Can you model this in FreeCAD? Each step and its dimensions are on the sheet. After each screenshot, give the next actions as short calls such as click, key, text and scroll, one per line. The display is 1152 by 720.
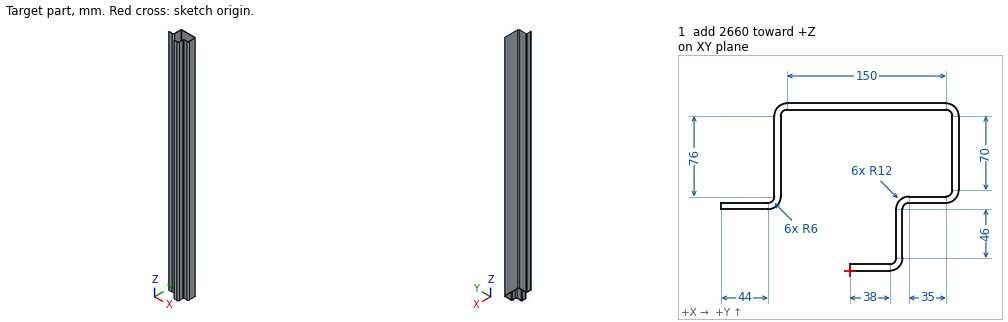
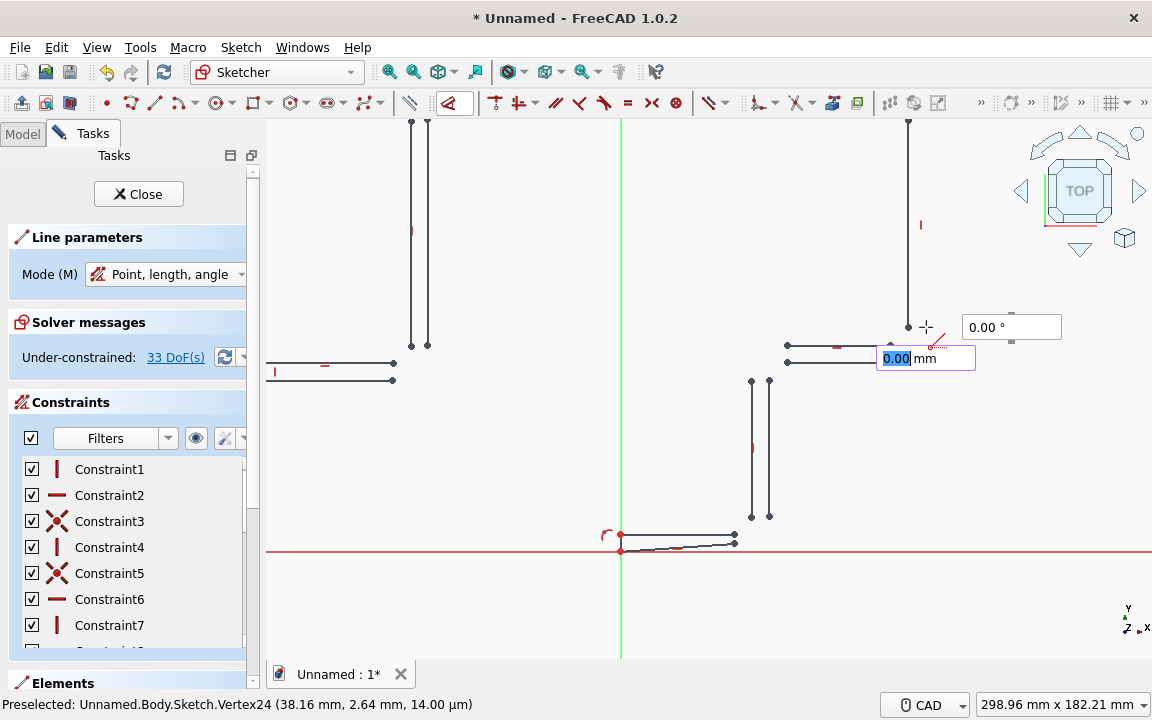
scroll(735, 534, down, 2)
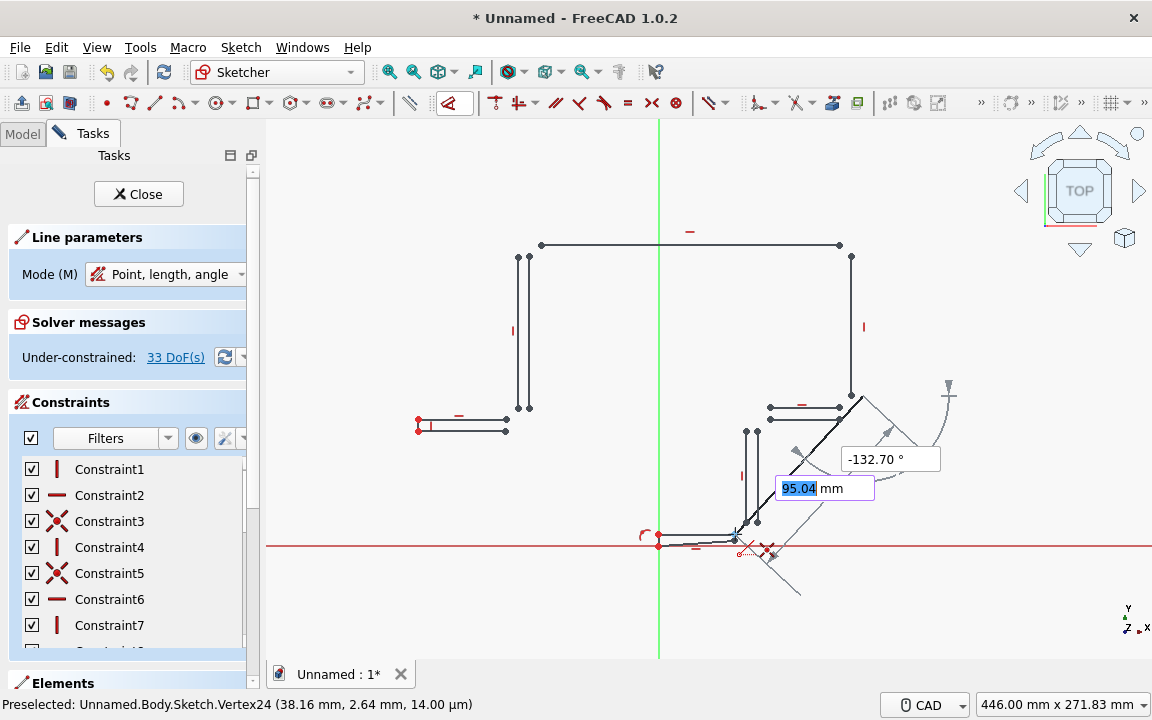
scroll(863, 256, up, 2)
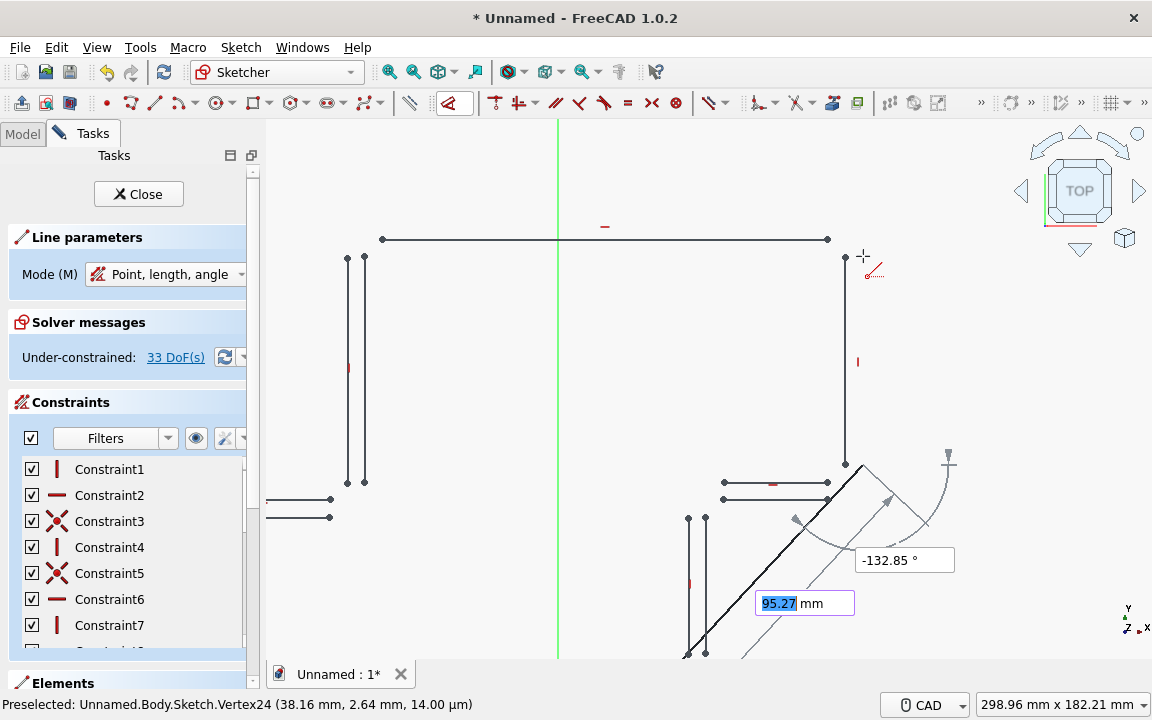
click(863, 256)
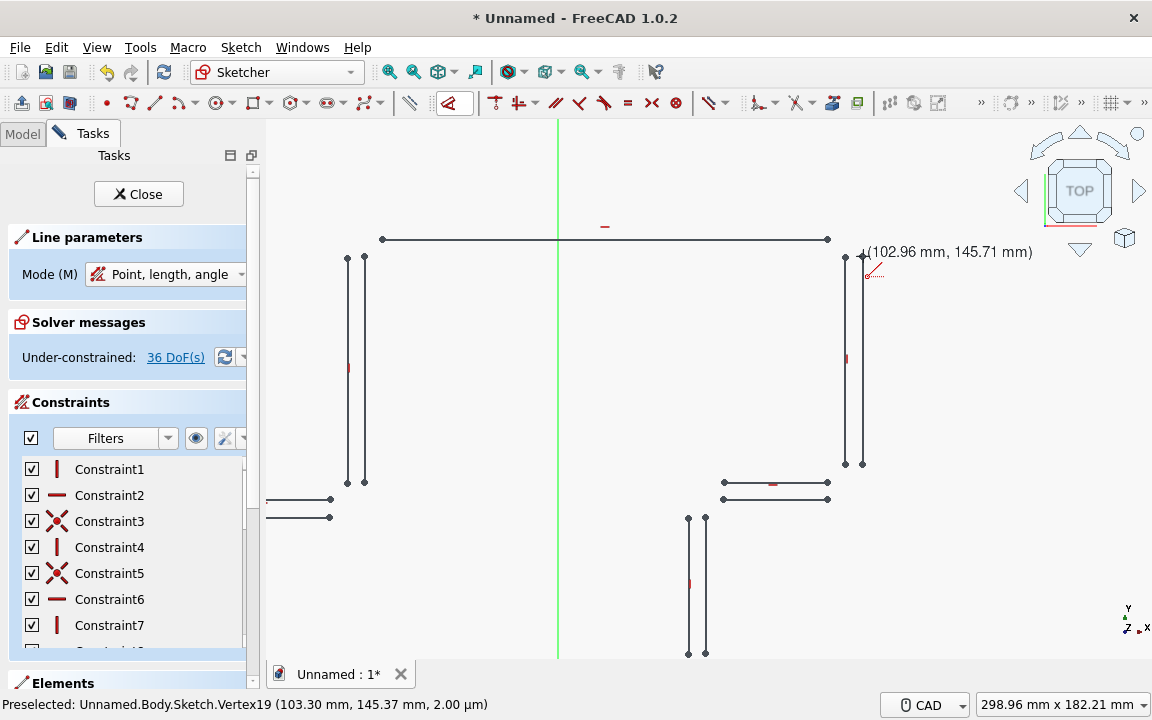
click(828, 221)
click(383, 221)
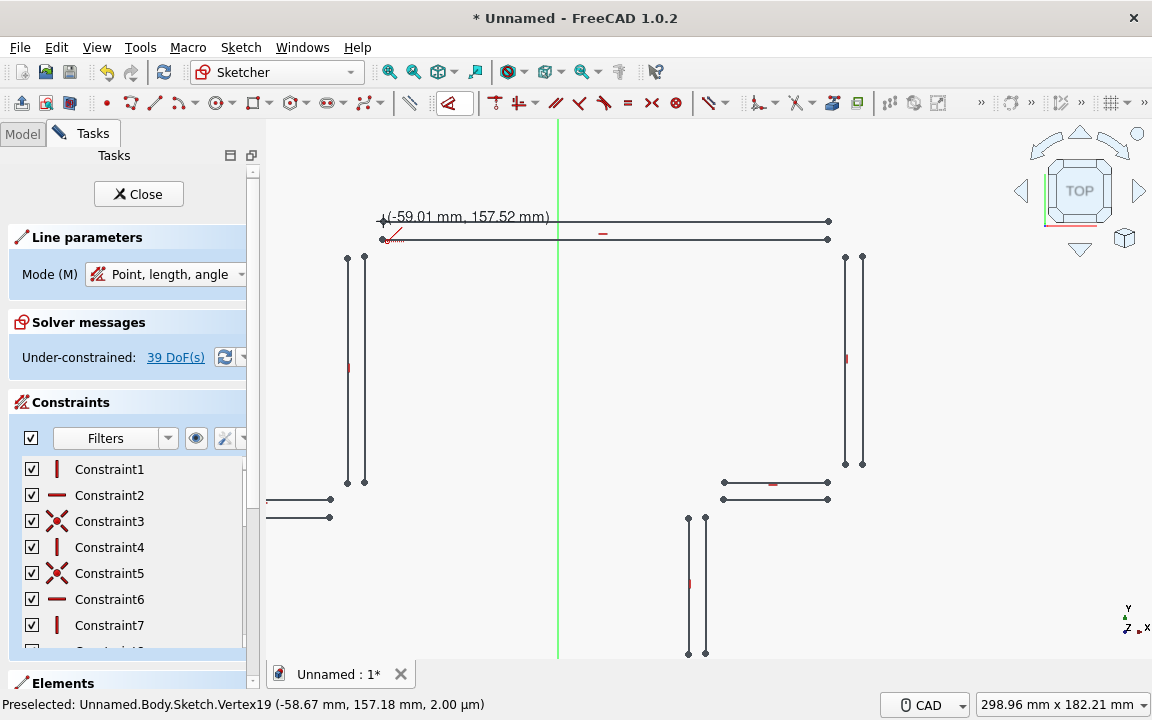
key(g)
key(3)
key(a)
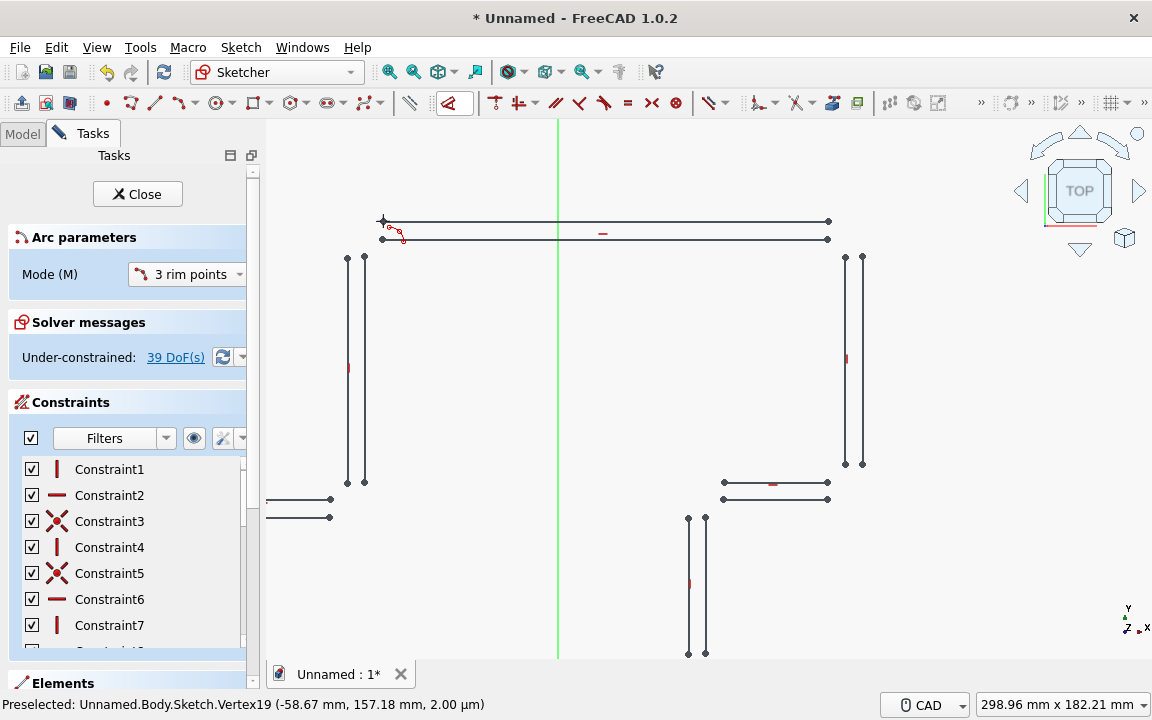
click(348, 484)
click(330, 500)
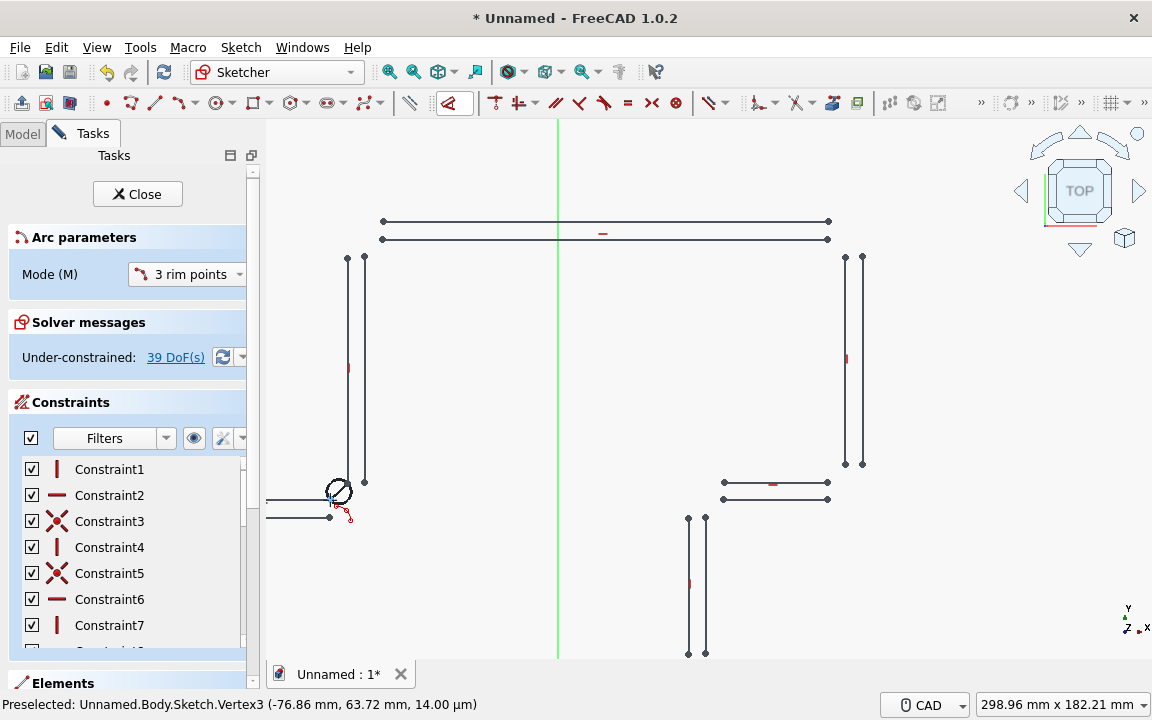
scroll(342, 494, up, 6)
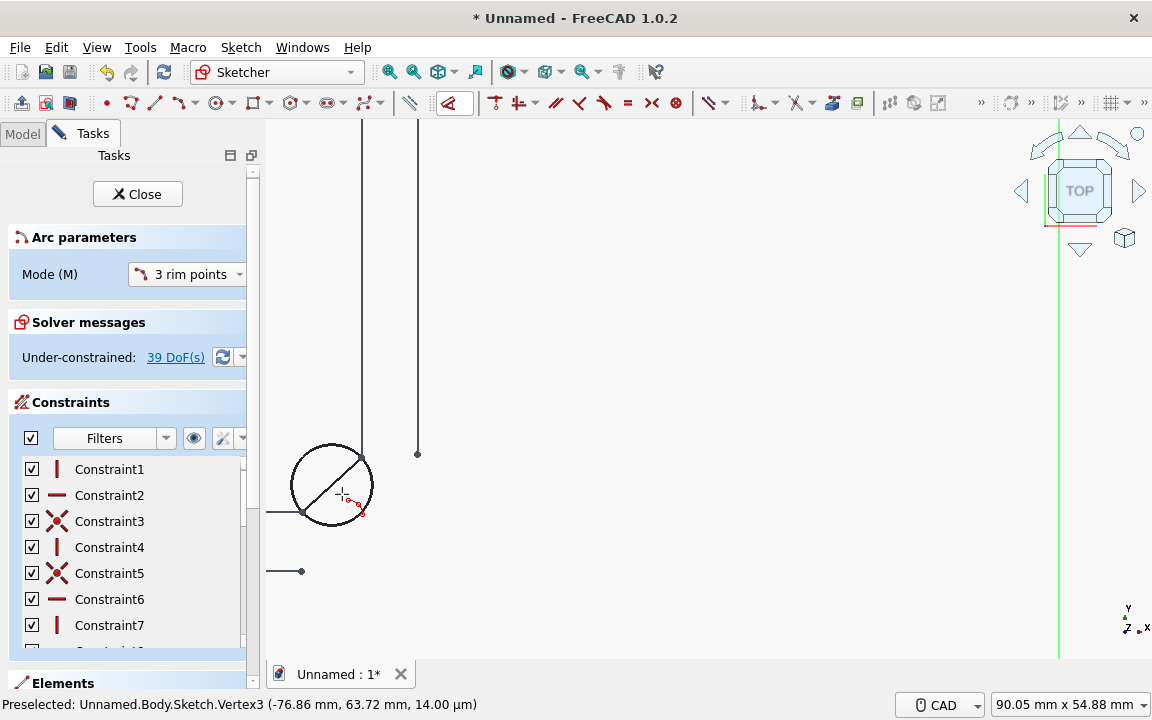
click(343, 492)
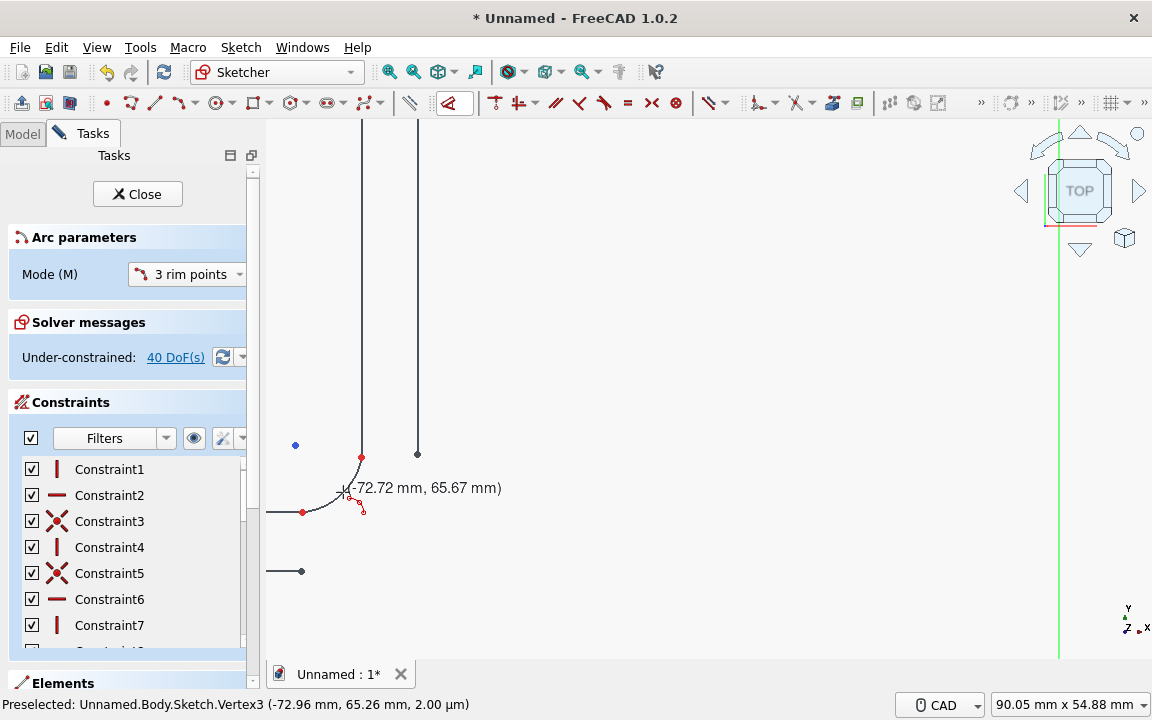
scroll(557, 396, down, 8)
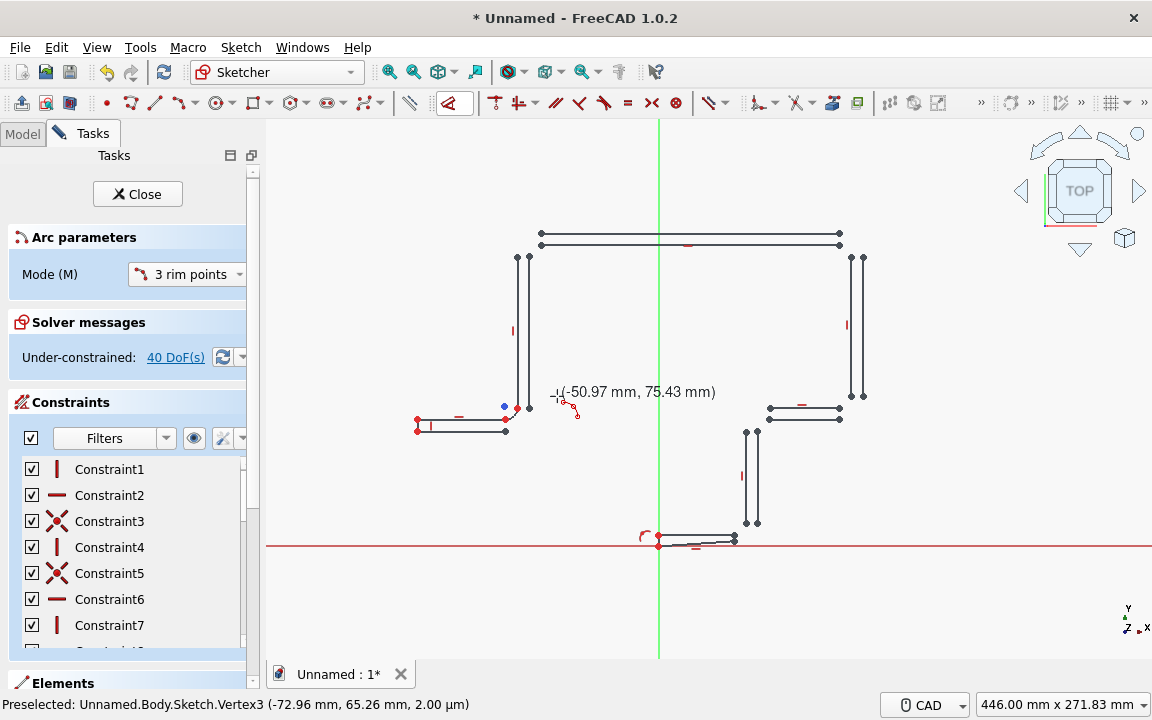
scroll(506, 431, up, 2)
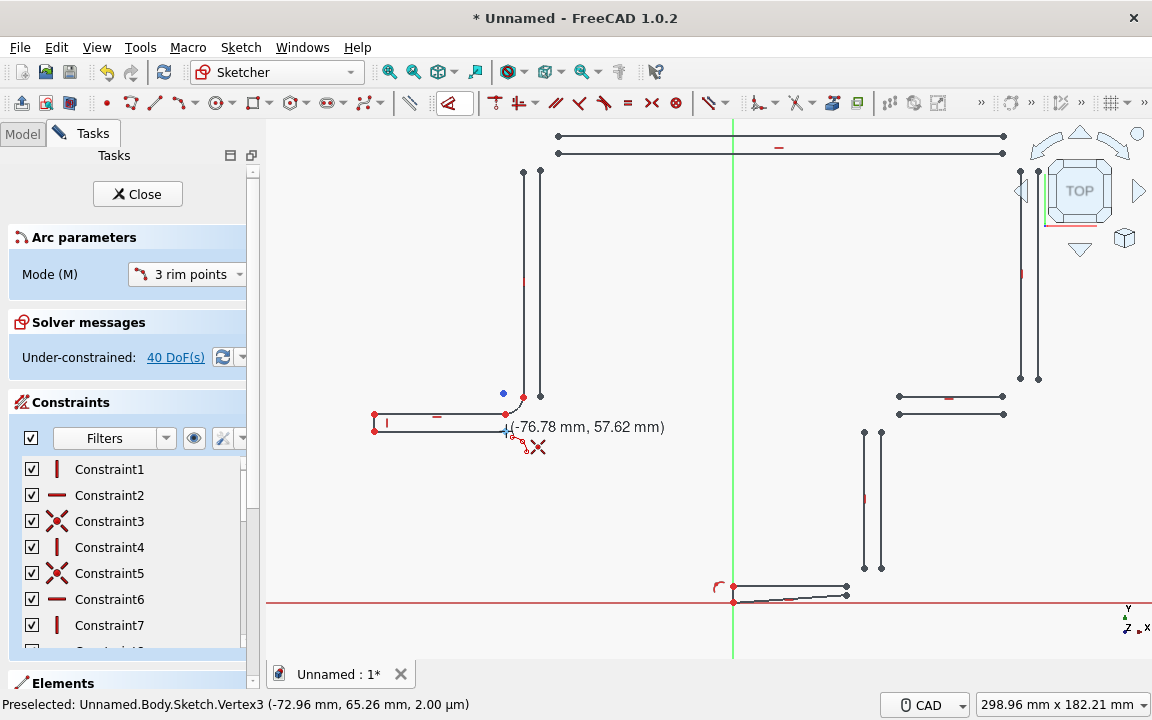
click(505, 432)
click(540, 397)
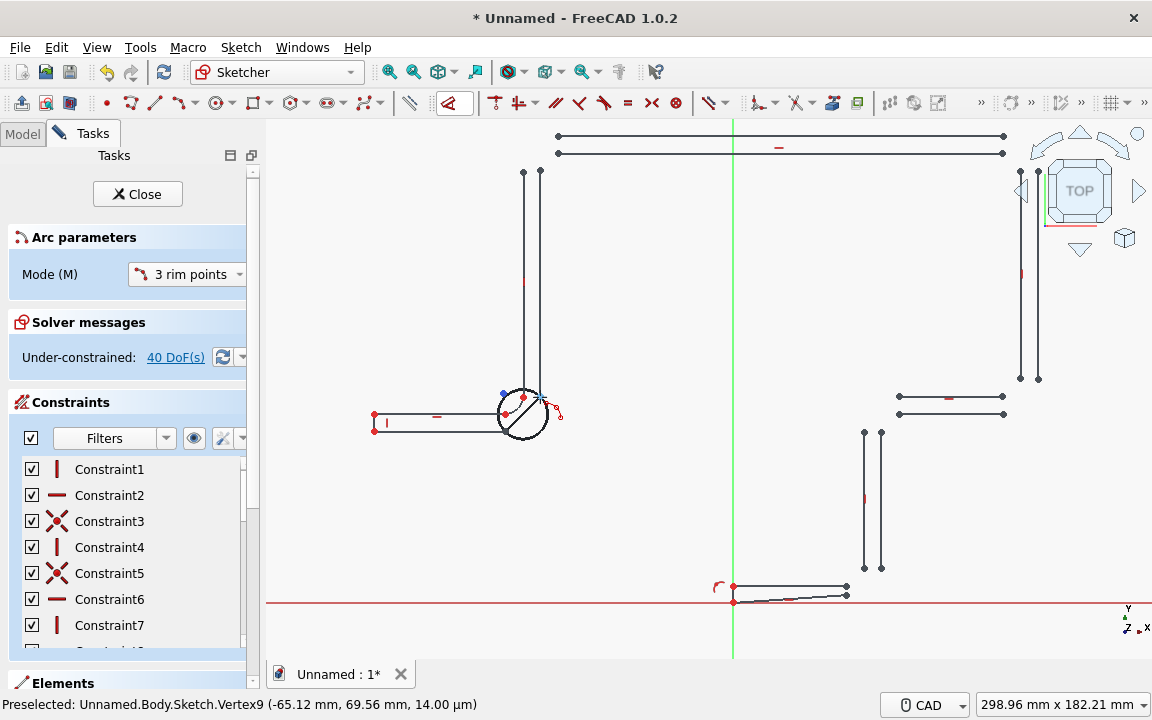
scroll(530, 421, up, 3)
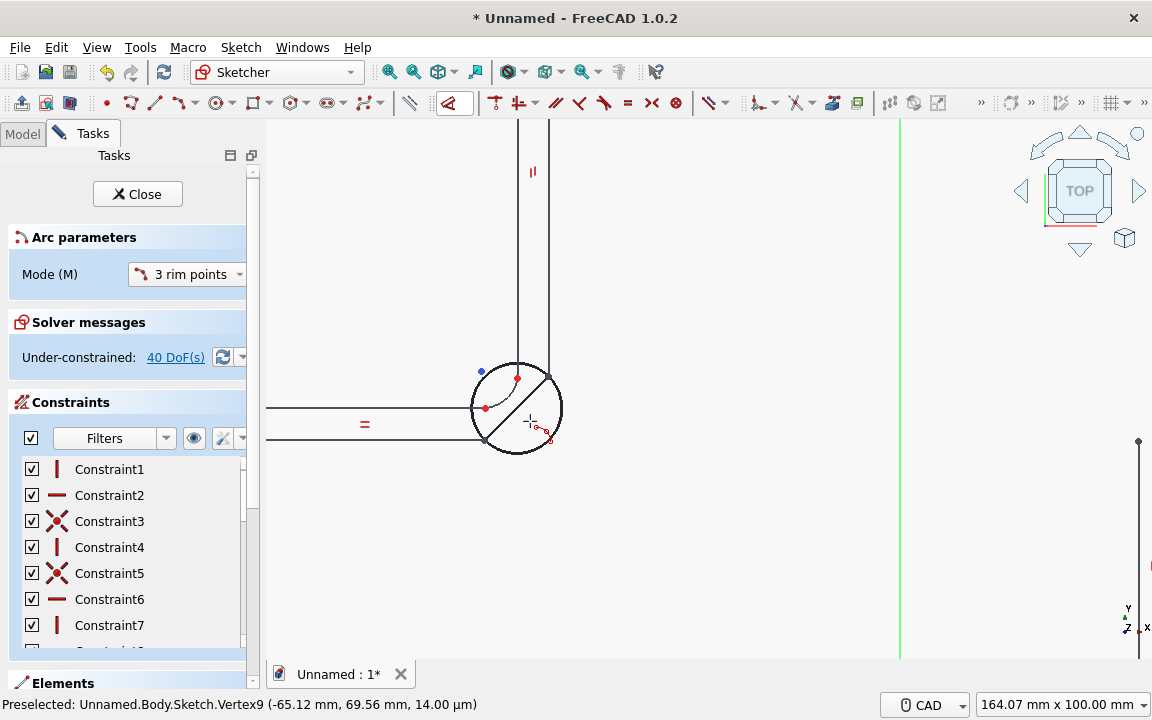
click(530, 420)